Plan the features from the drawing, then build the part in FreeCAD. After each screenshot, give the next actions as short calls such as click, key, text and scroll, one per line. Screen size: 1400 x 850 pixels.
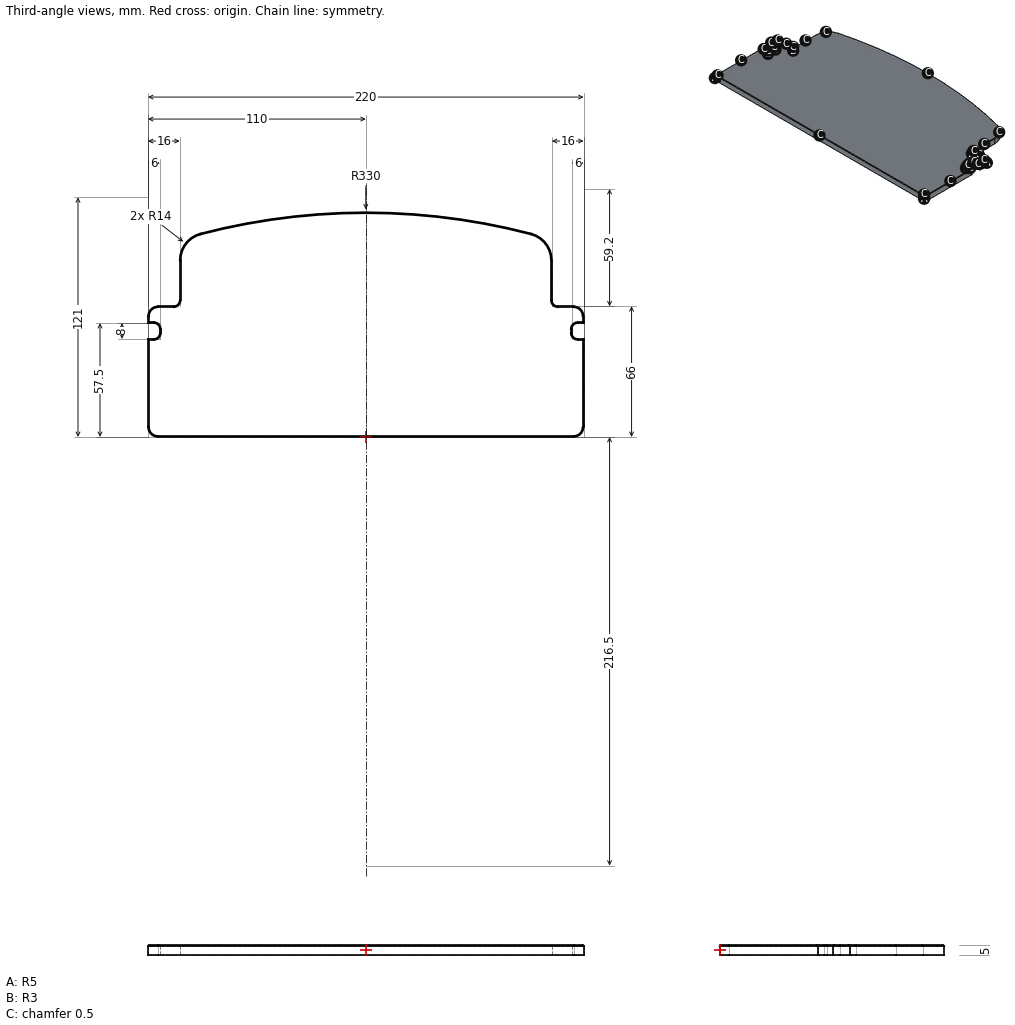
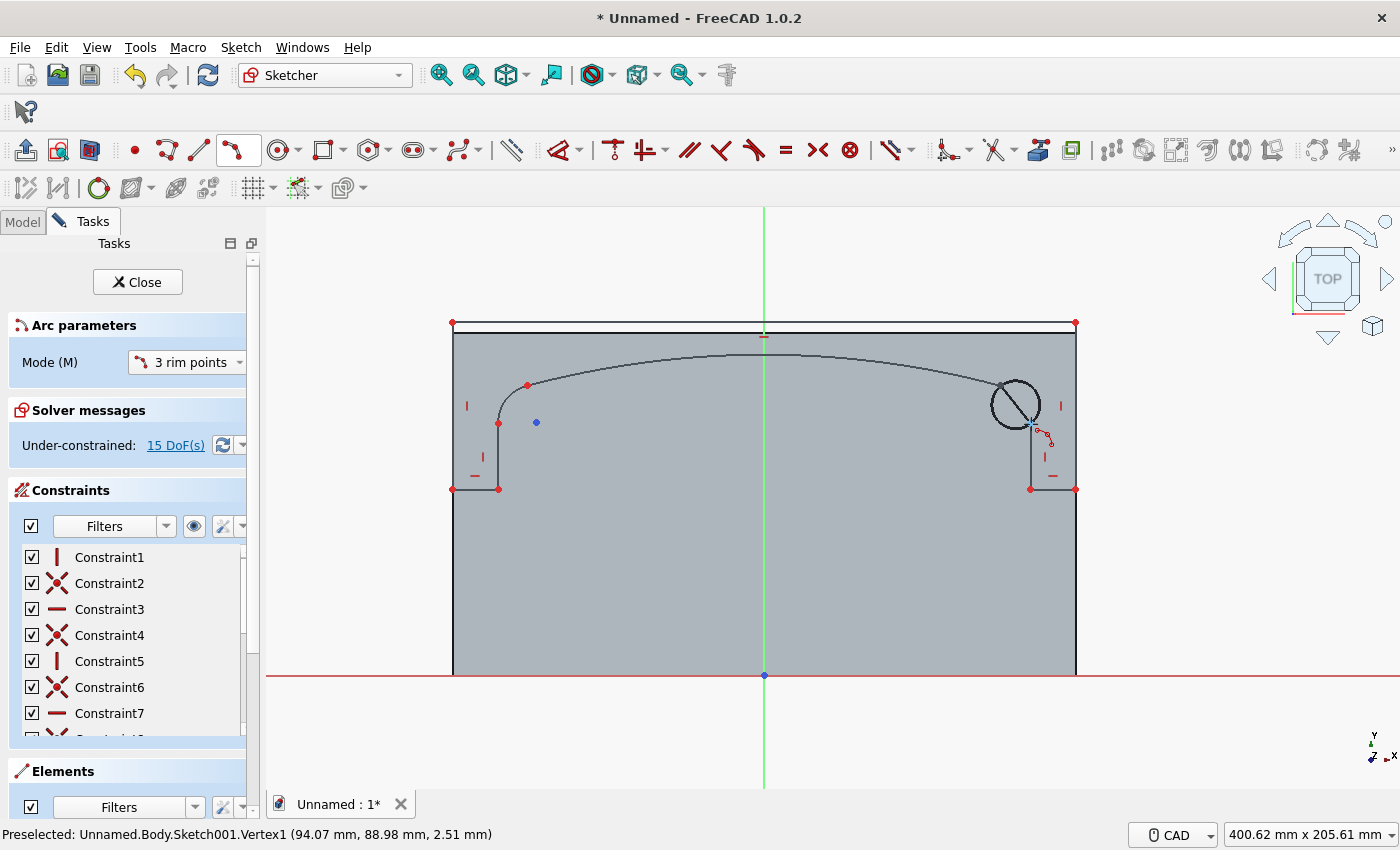
scroll(1022, 399, up, 4)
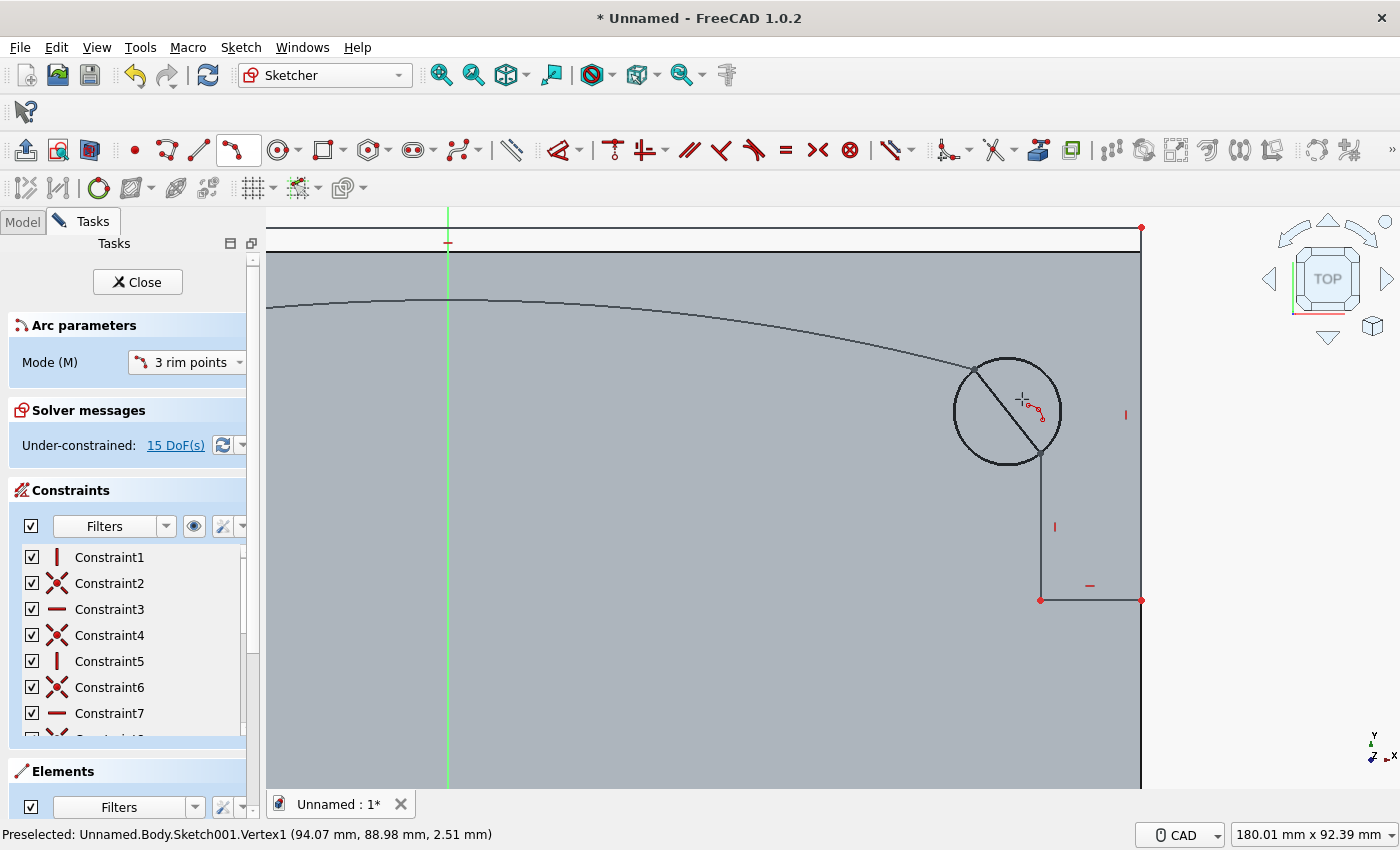
click(1022, 398)
key(Escape)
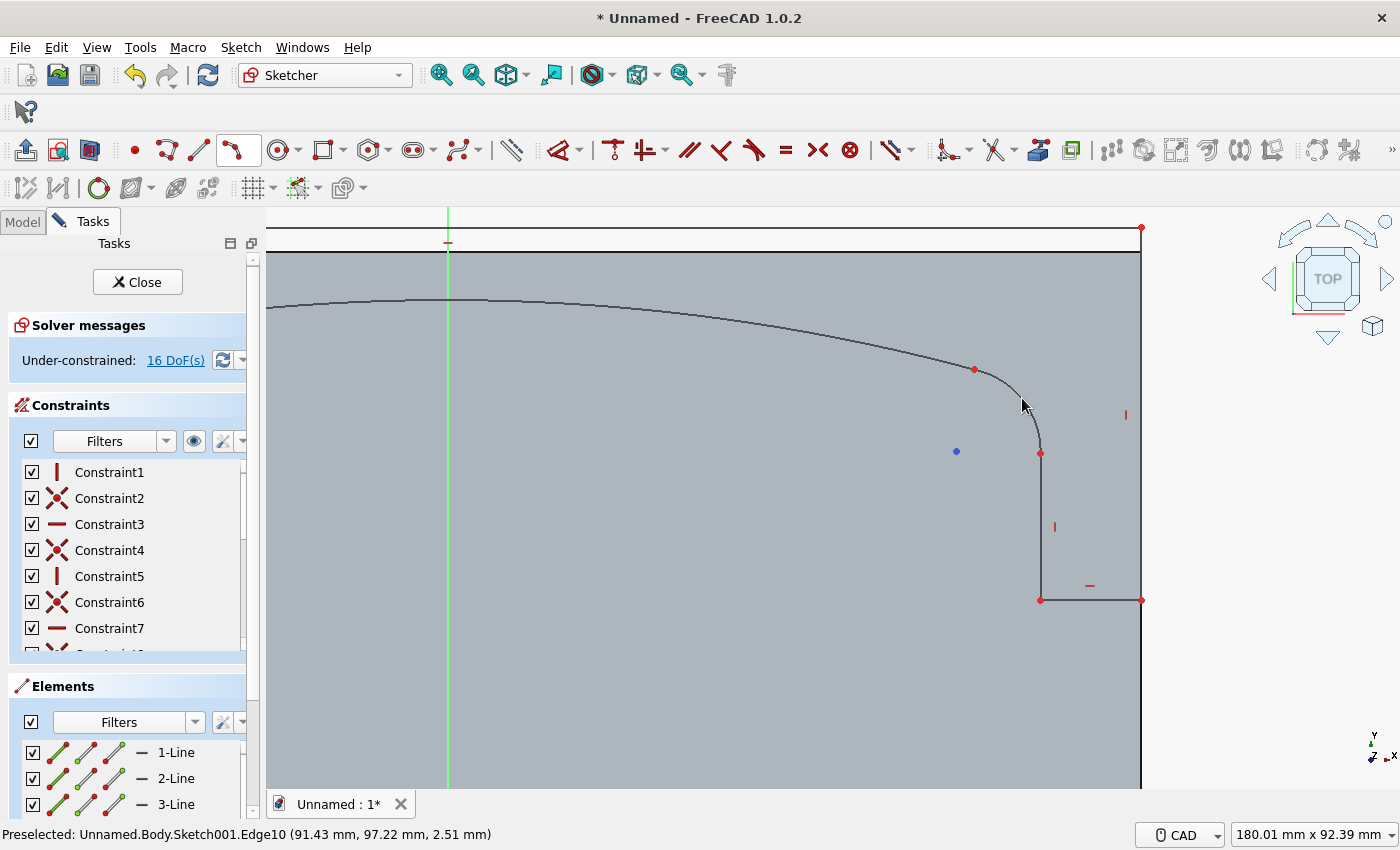
click(1041, 498)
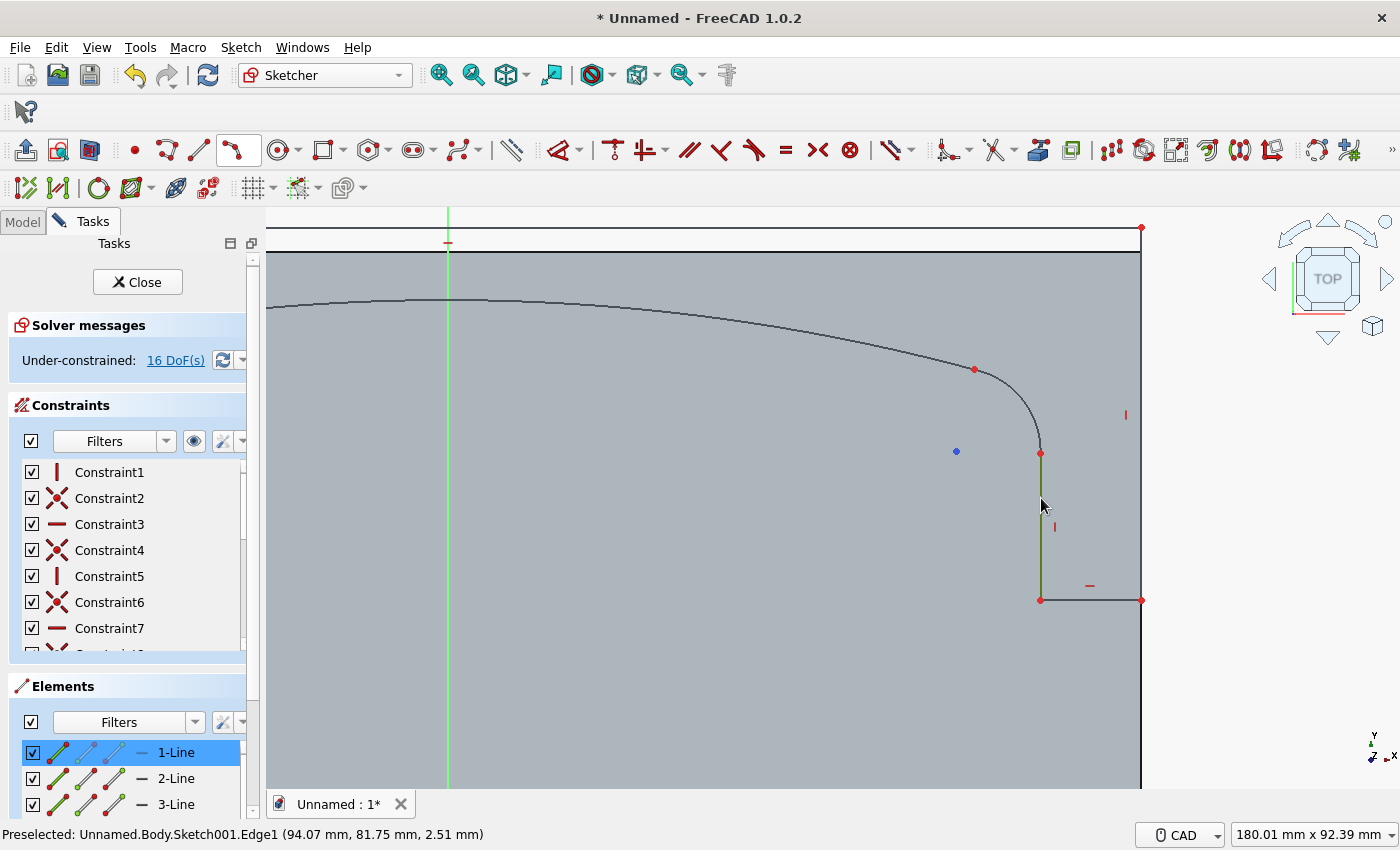
click(1034, 420)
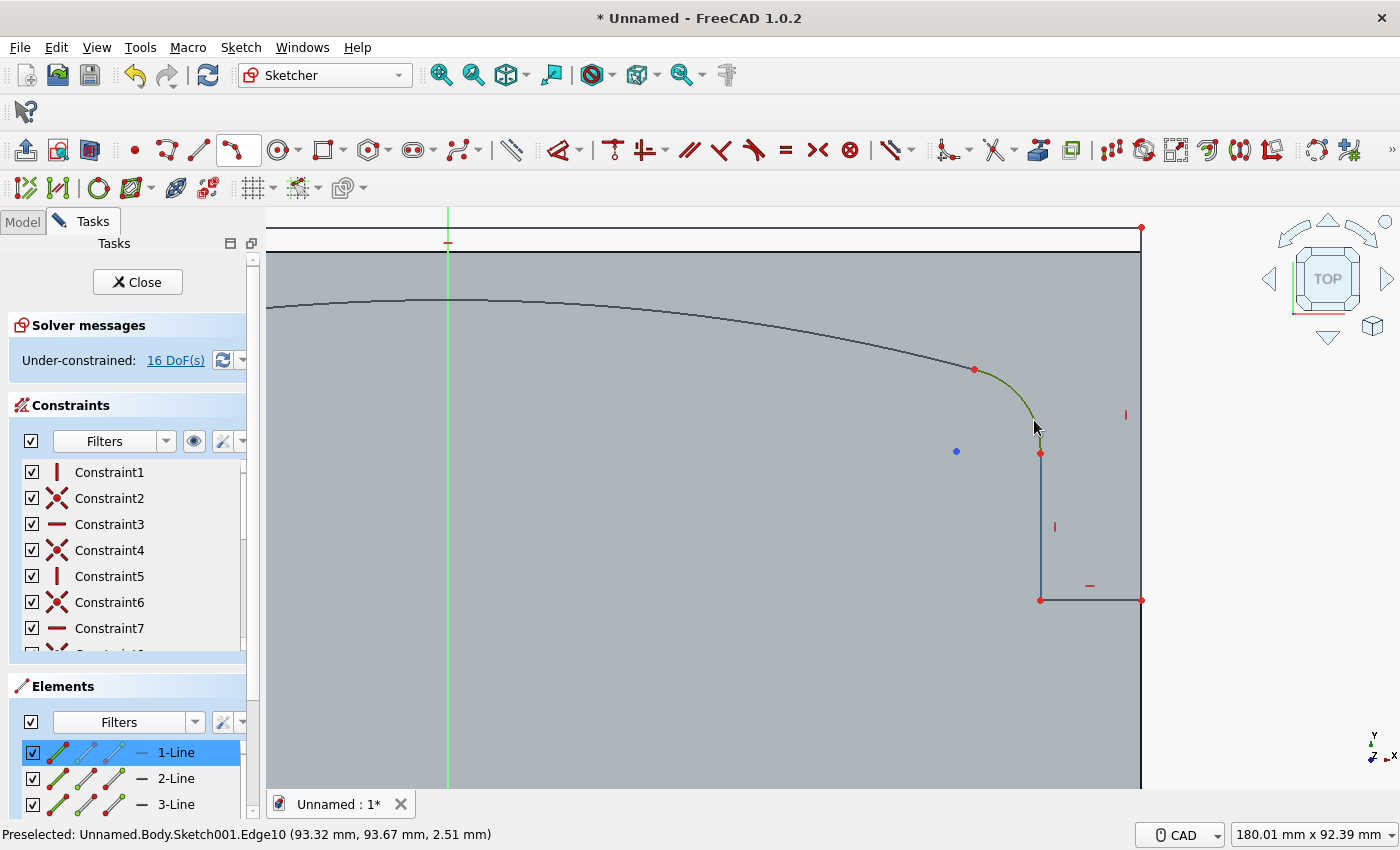
key(t)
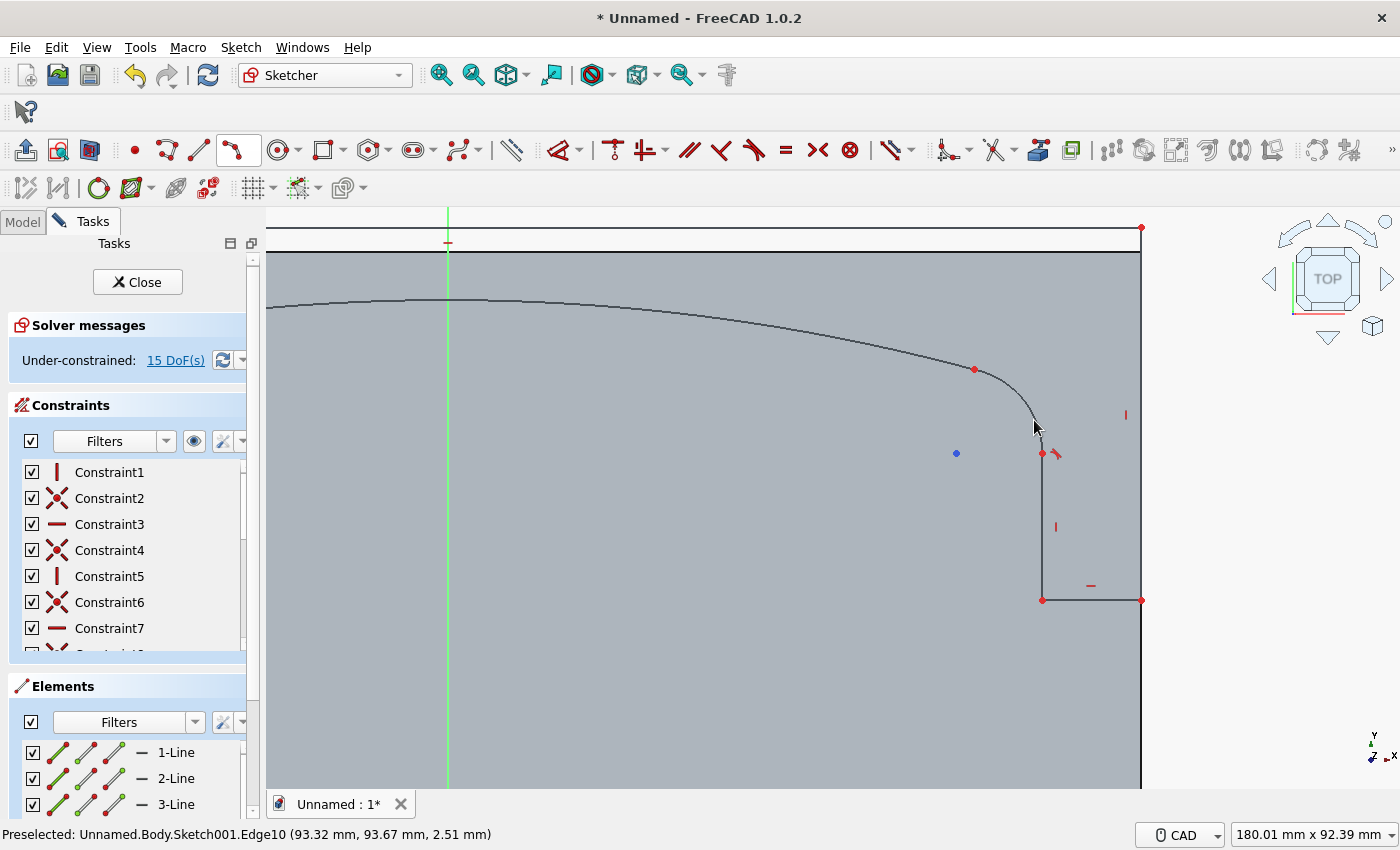
scroll(1023, 399, down, 4)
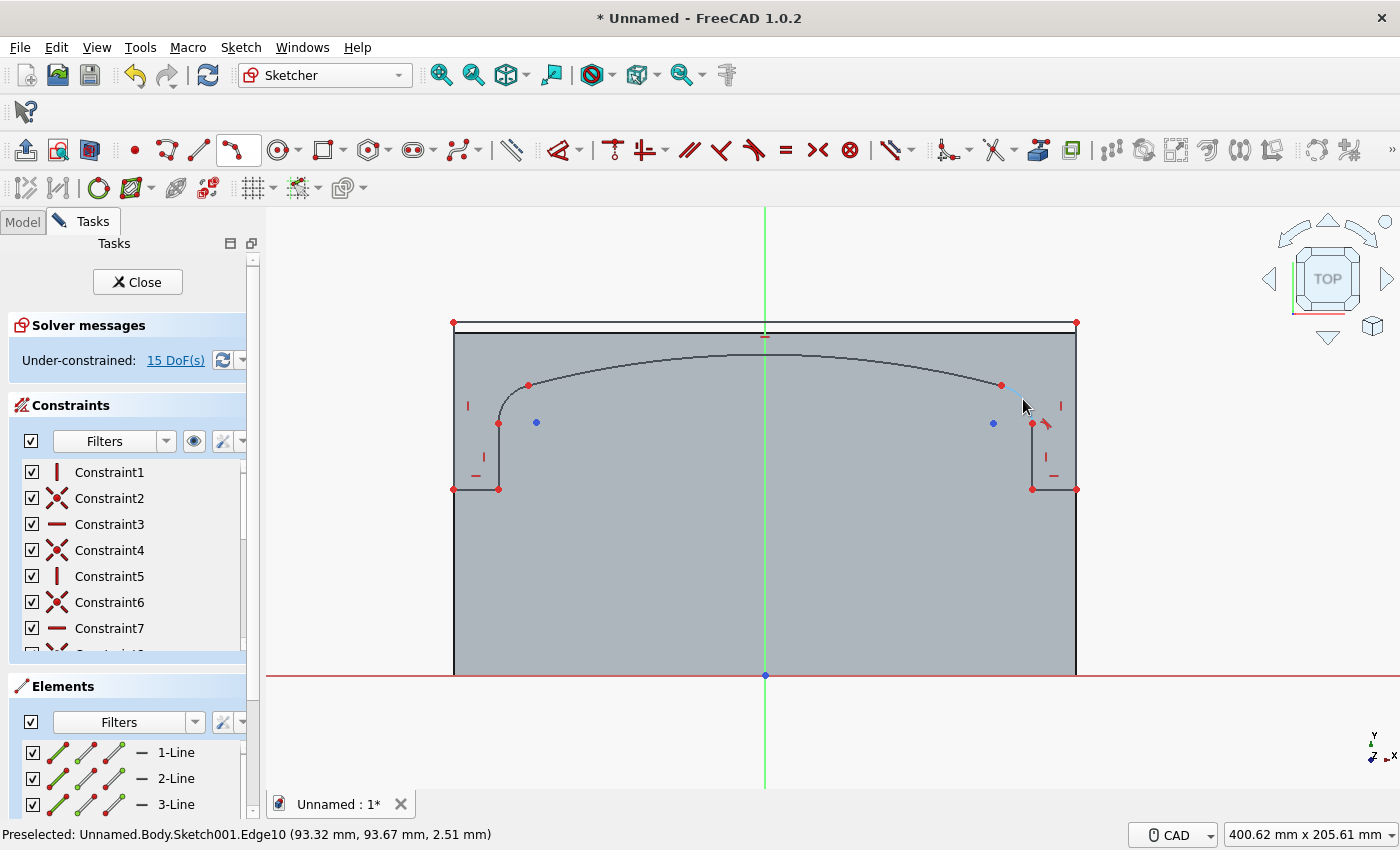
click(499, 470)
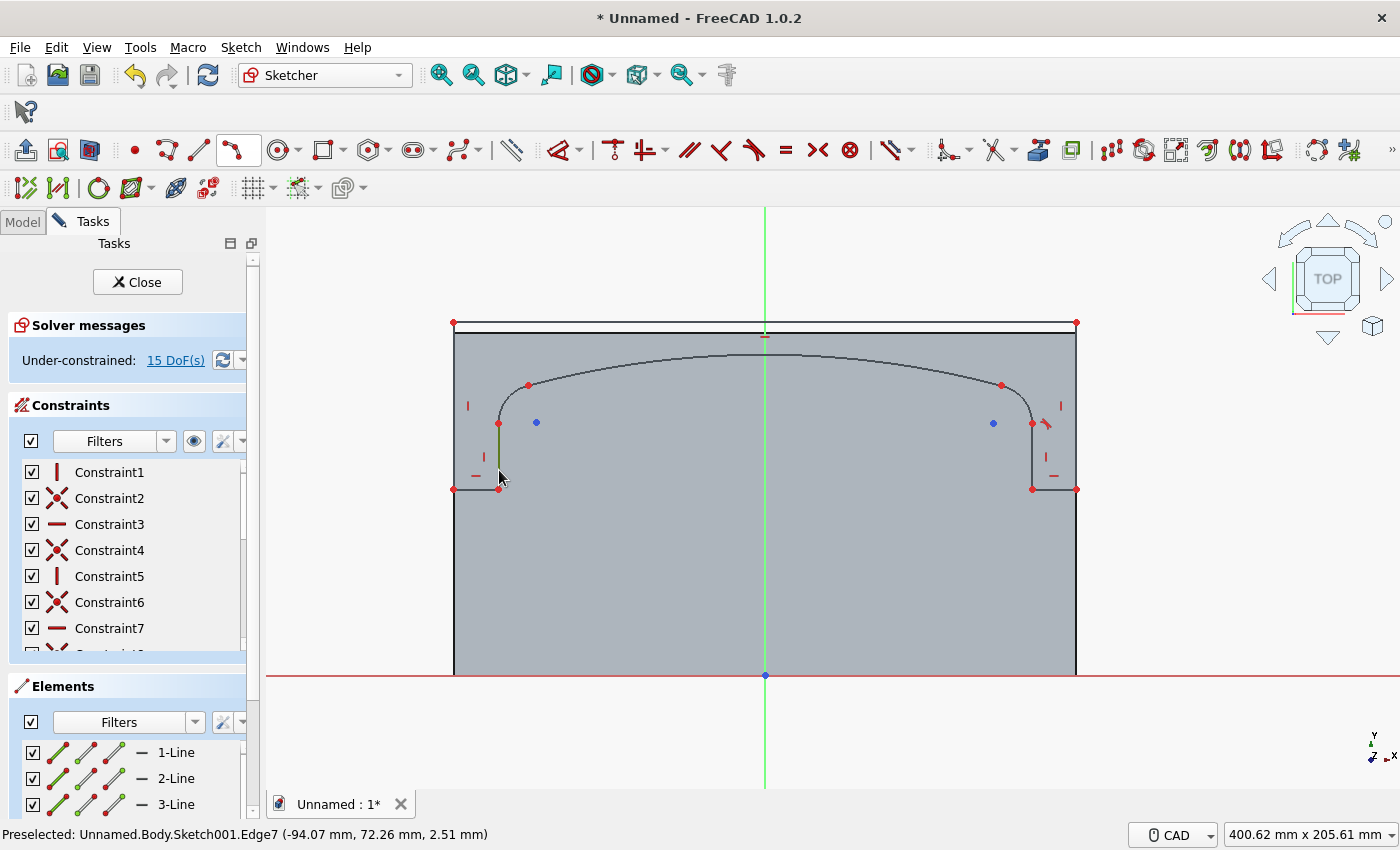
click(514, 392)